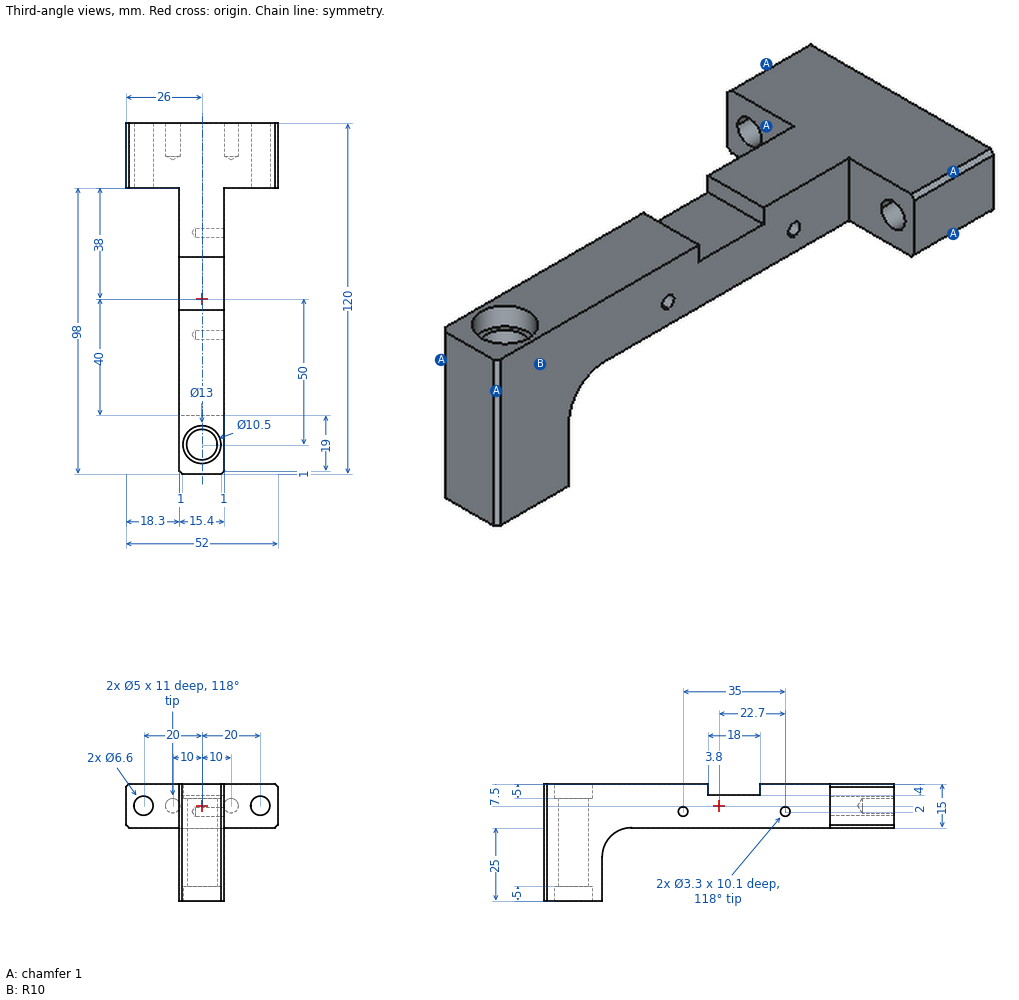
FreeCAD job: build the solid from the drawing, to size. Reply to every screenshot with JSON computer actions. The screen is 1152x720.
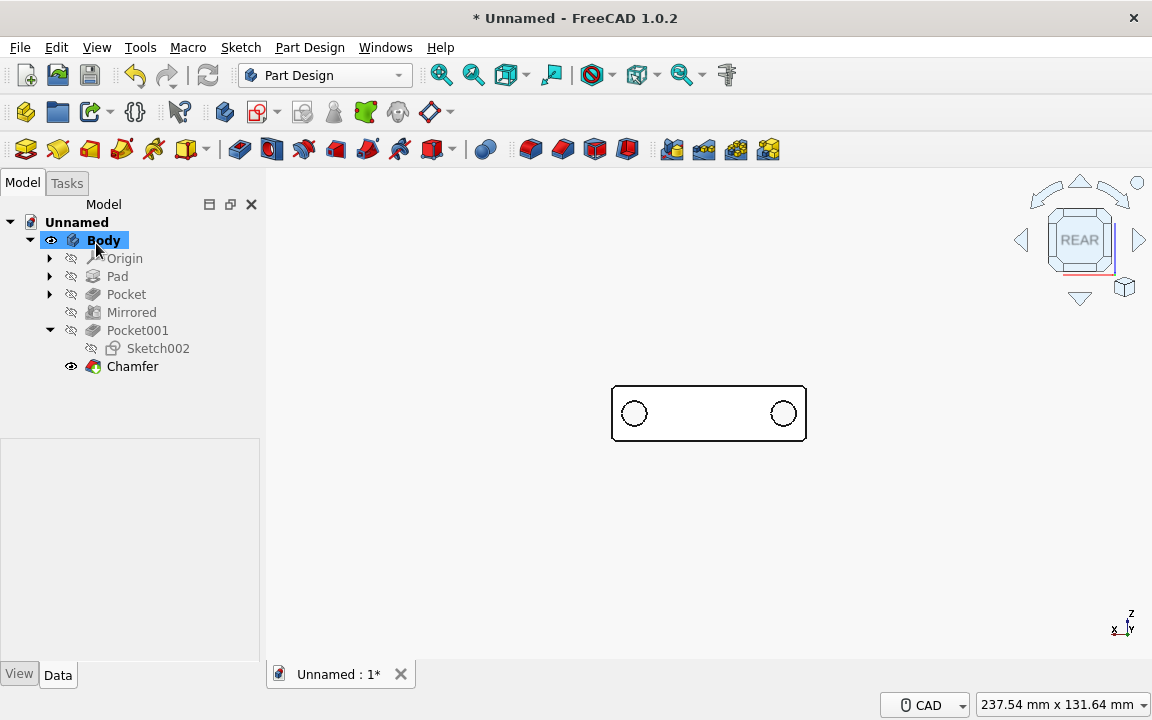
{"action": "left_click", "coordinate": [442, 76]}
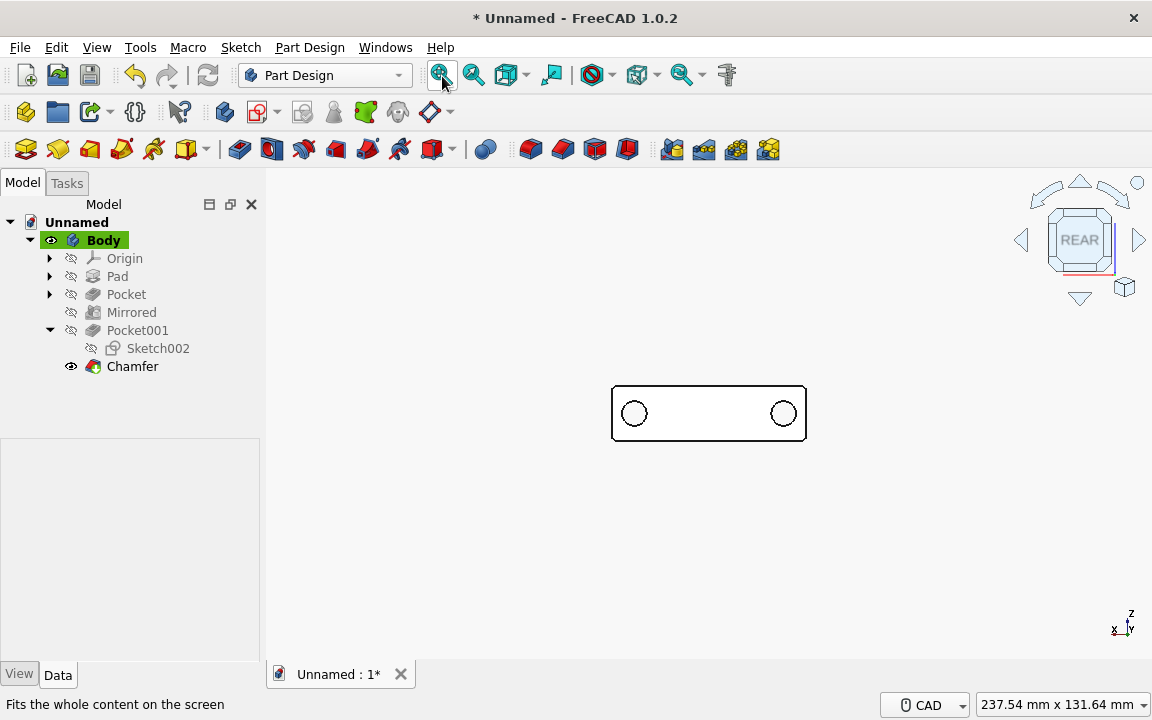
{"action": "left_click", "coordinate": [681, 413]}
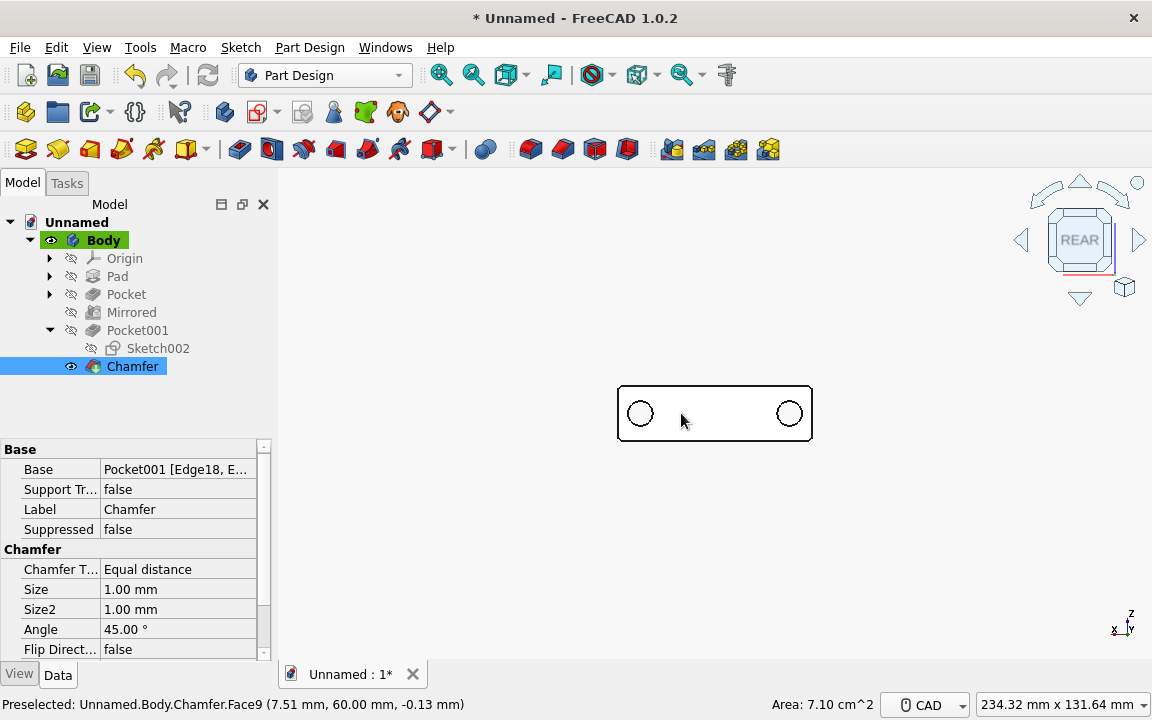
{"action": "left_click", "coordinate": [258, 112]}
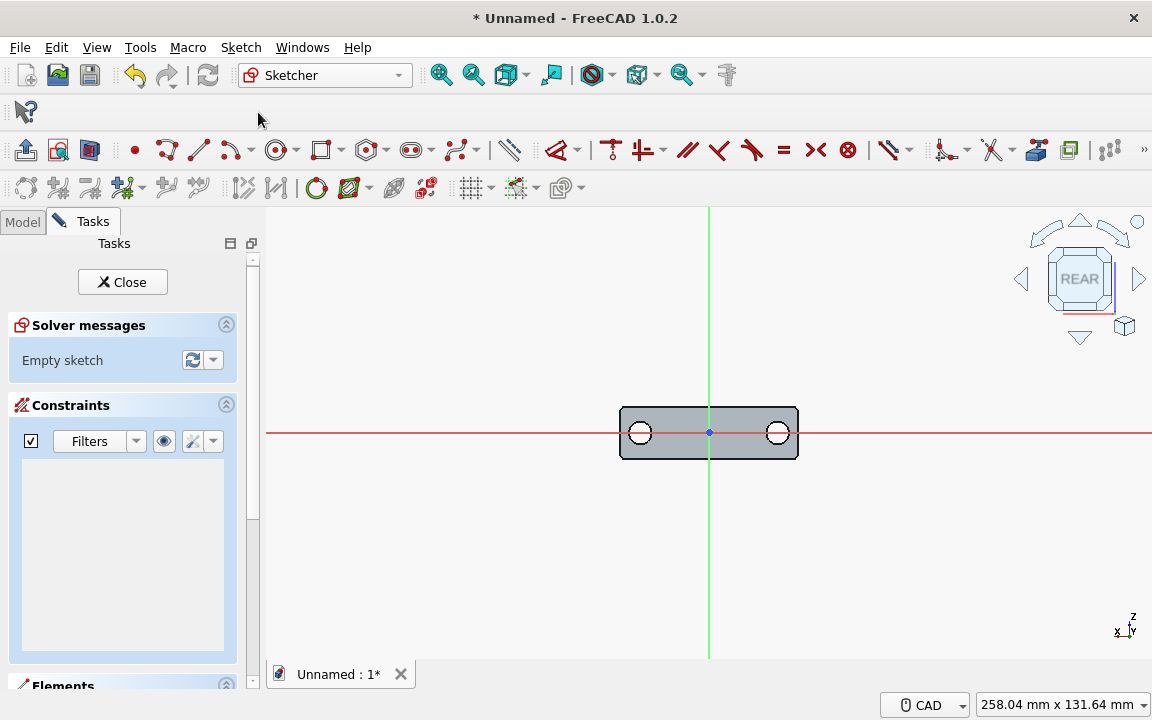
{"action": "scroll", "coordinate": [723, 433], "scroll_direction": "up", "scroll_amount": 9}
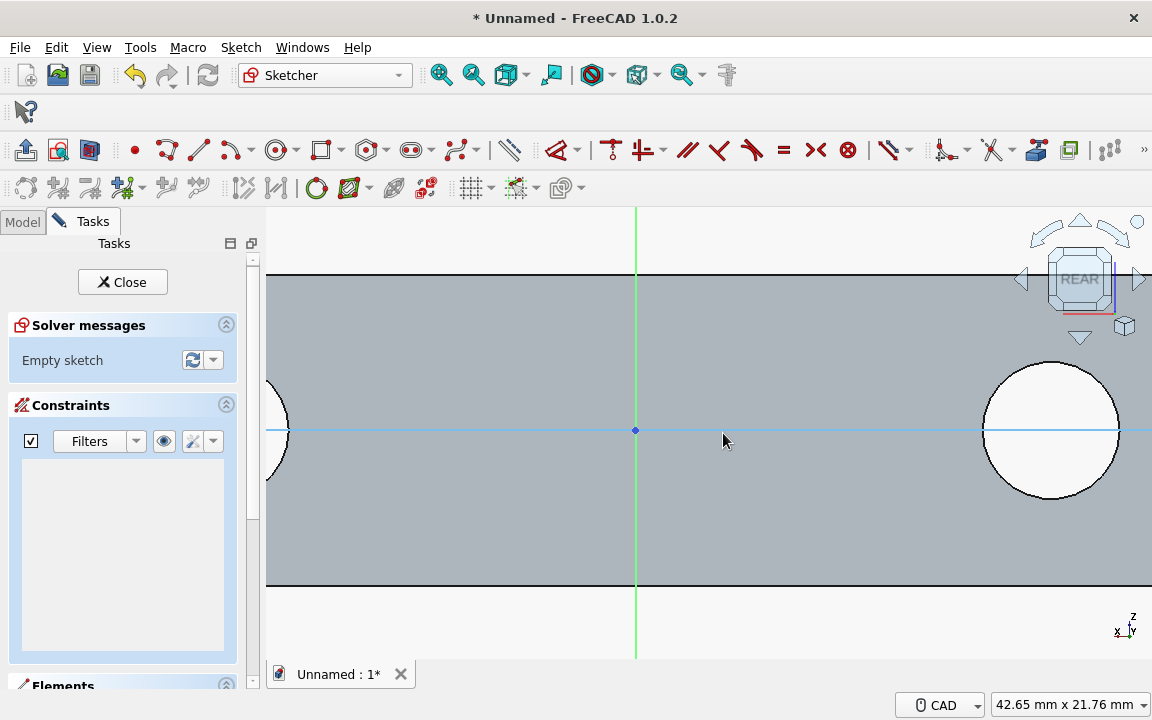
{"action": "left_click", "coordinate": [276, 150]}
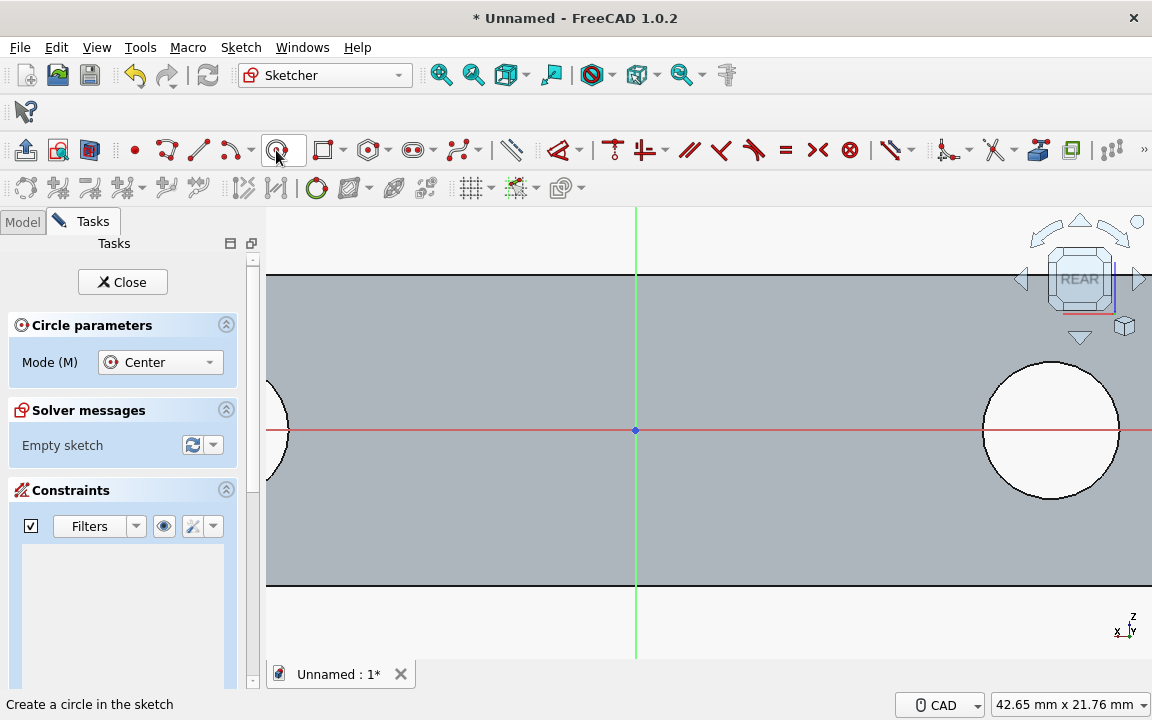
{"action": "left_click", "coordinate": [843, 430]}
{"action": "mouse_move", "coordinate": [880, 394]}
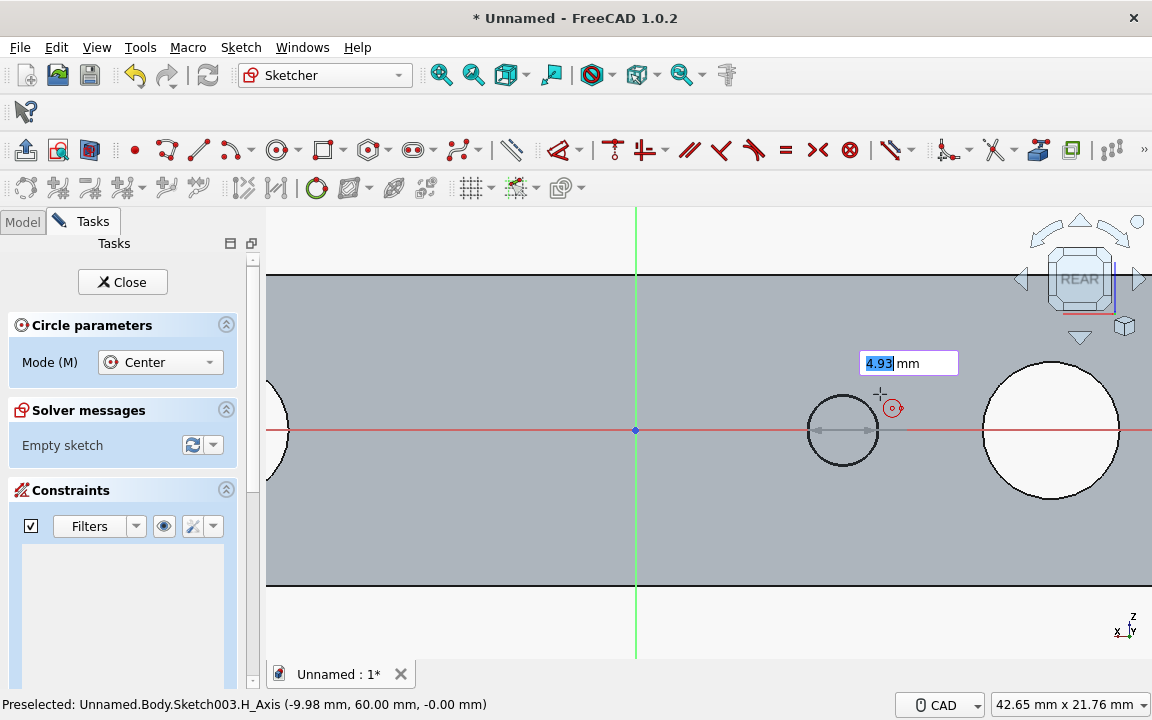
{"action": "type", "text": "5"}
{"action": "key", "text": "Return"}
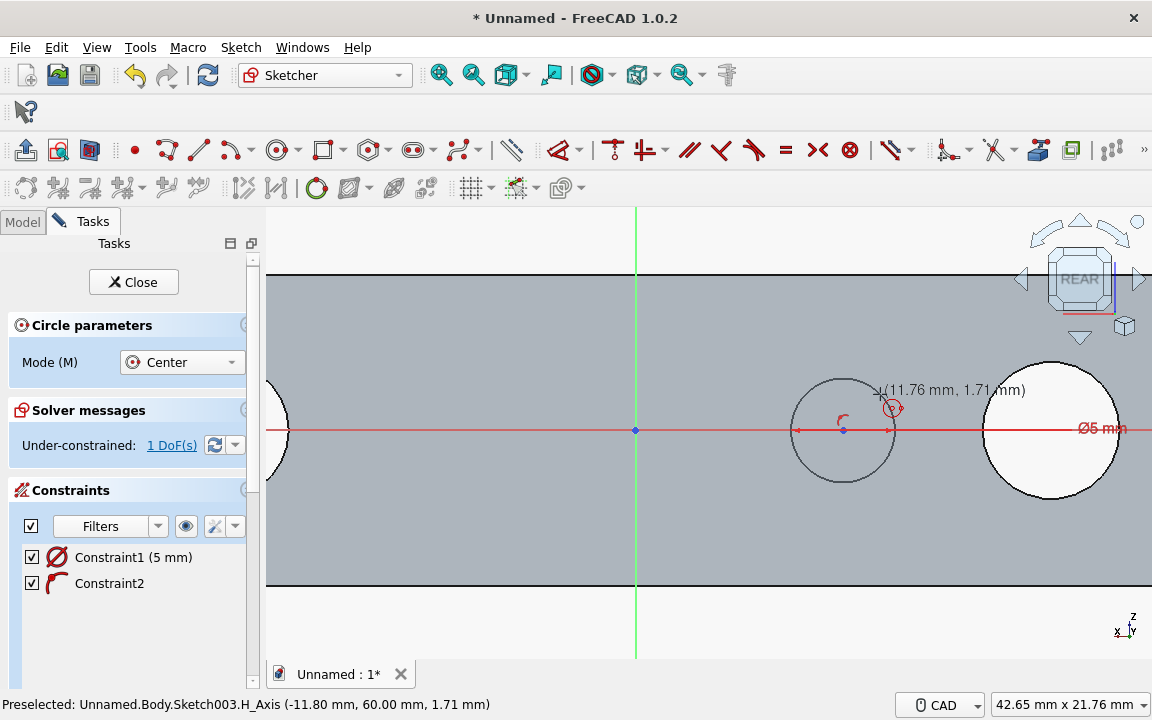
{"action": "left_click", "coordinate": [428, 430]}
{"action": "mouse_move", "coordinate": [465, 394]}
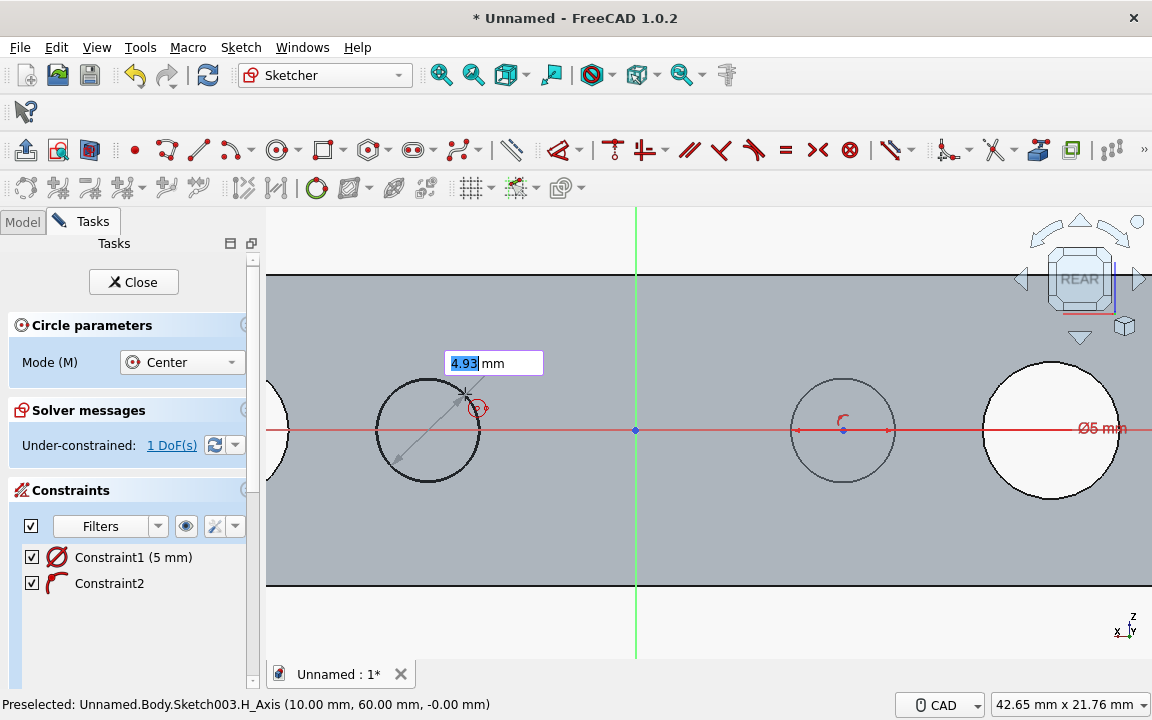
{"action": "type", "text": "5"}
{"action": "key", "text": "Return"}
{"action": "key", "text": "Escape"}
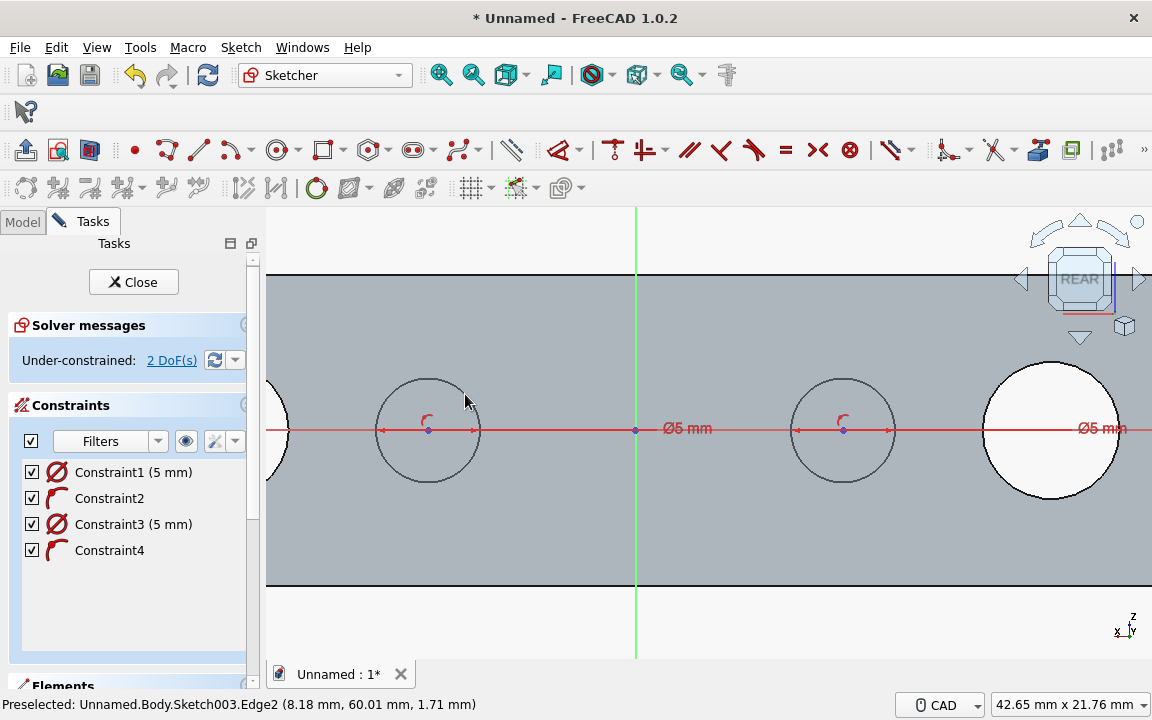
{"action": "left_click", "coordinate": [558, 150]}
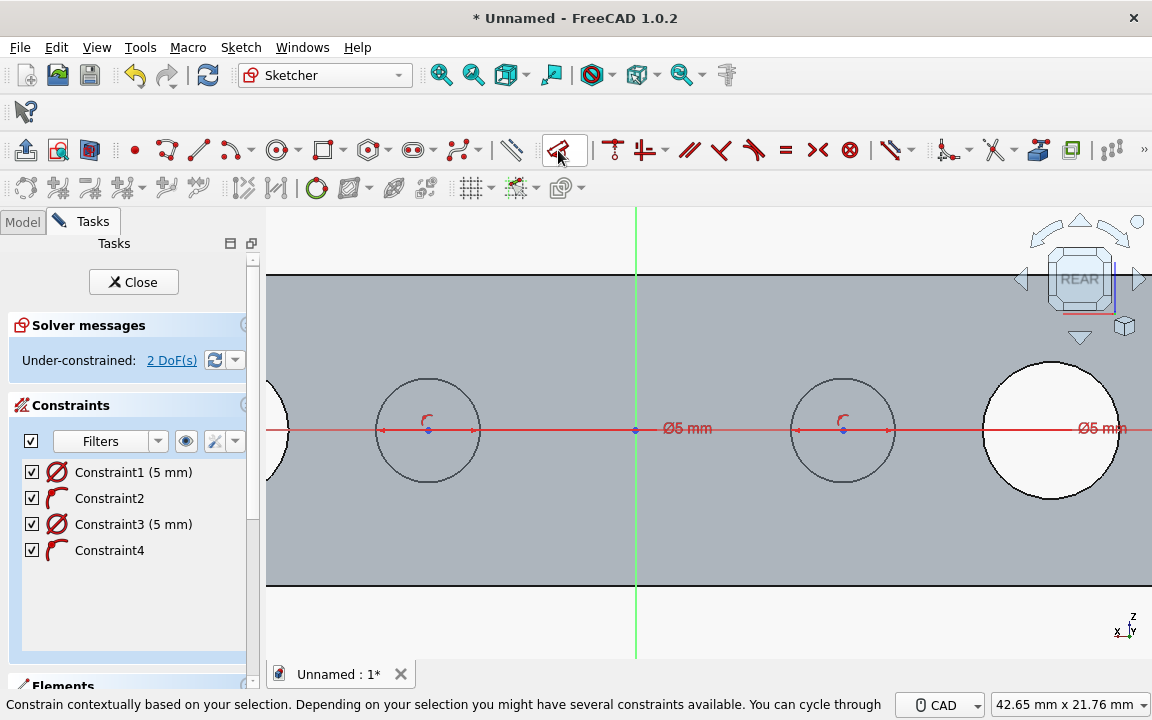
{"action": "left_click", "coordinate": [843, 430]}
{"action": "left_click", "coordinate": [739, 464]}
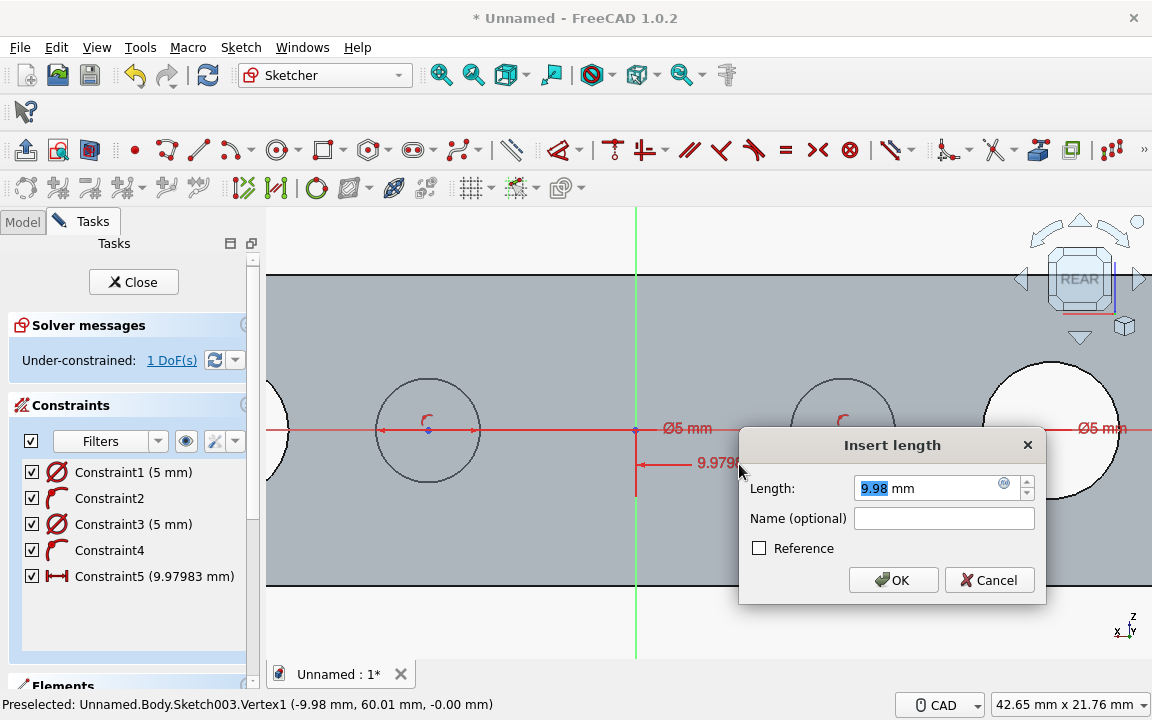
{"action": "type", "text": "10"}
{"action": "key", "text": "Return"}